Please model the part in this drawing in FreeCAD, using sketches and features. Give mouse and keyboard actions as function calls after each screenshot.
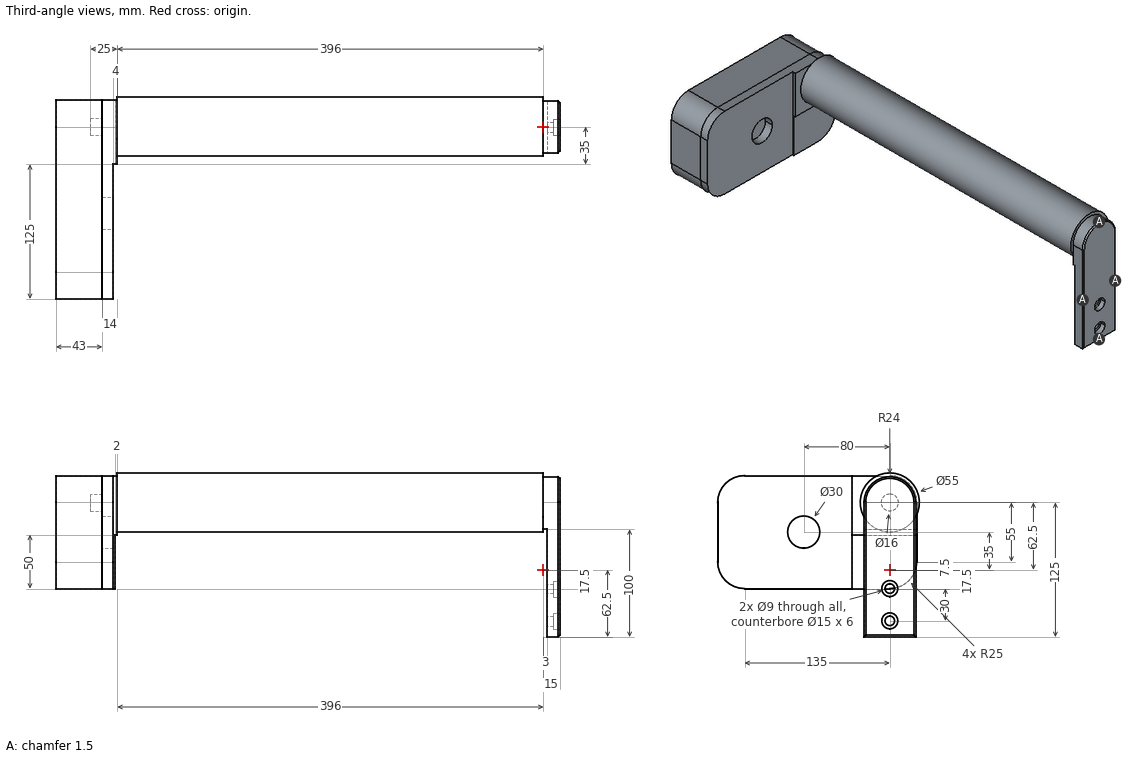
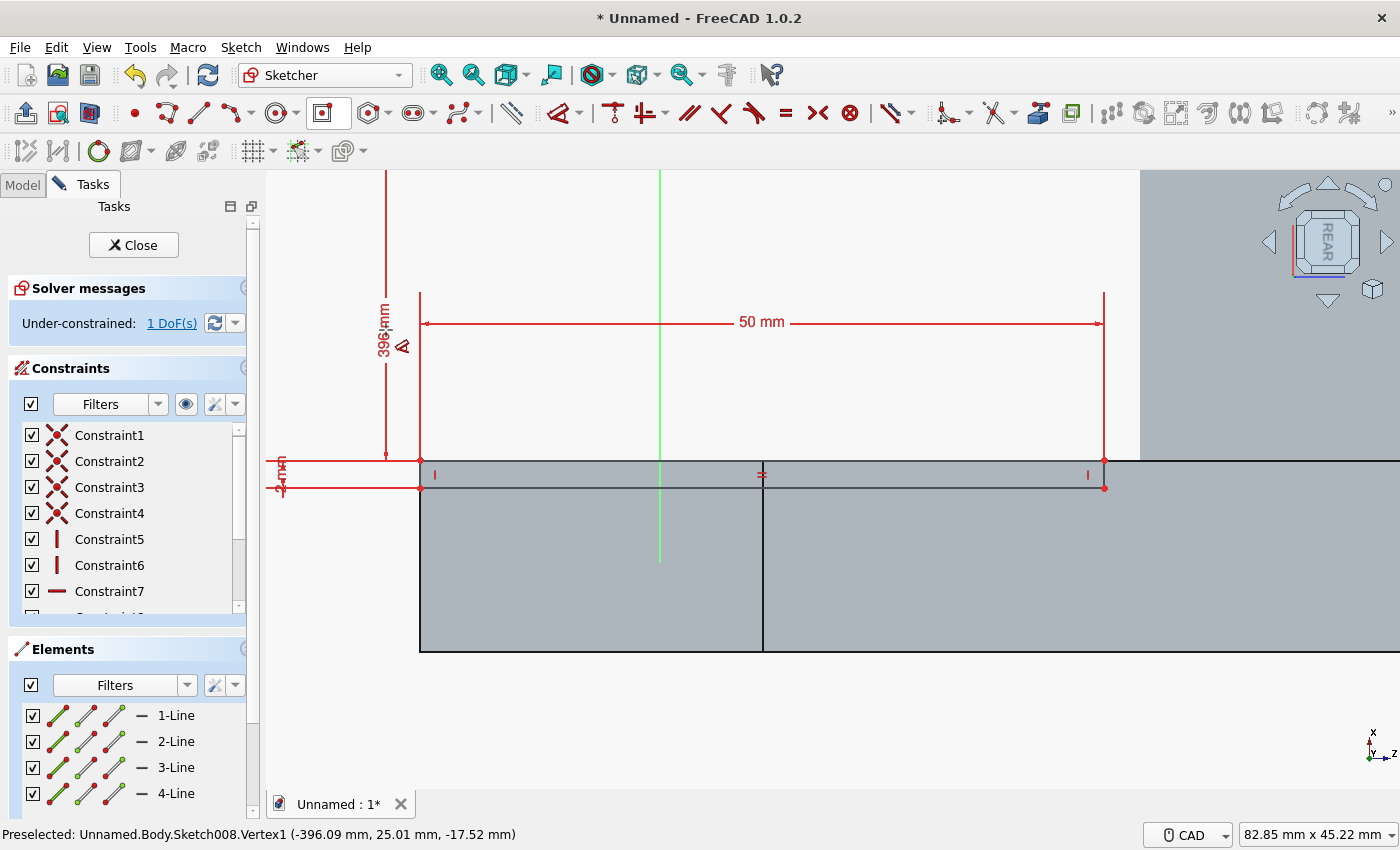
click(420, 461)
click(540, 519)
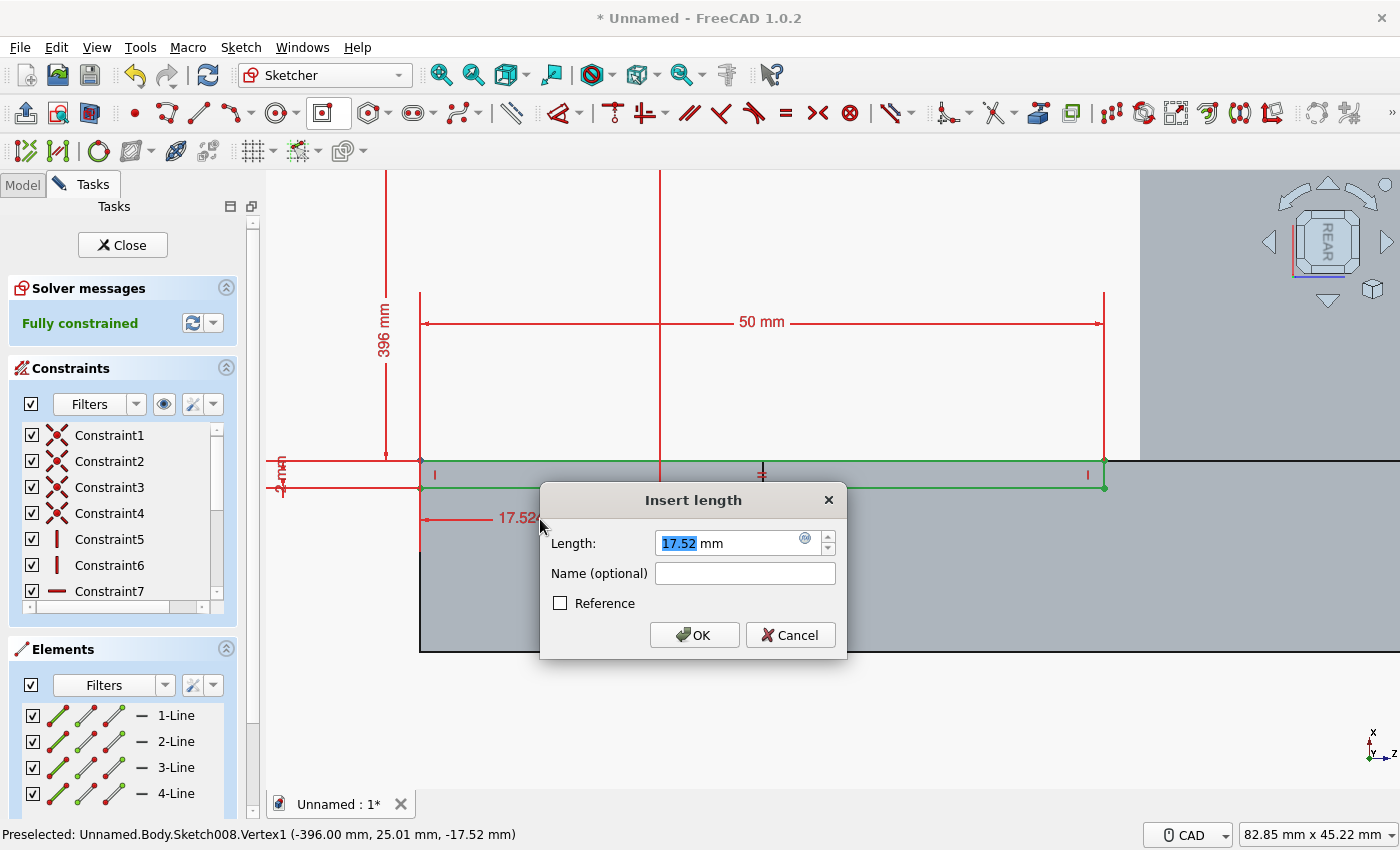
text(17.5)
key(Return)
key(Escape)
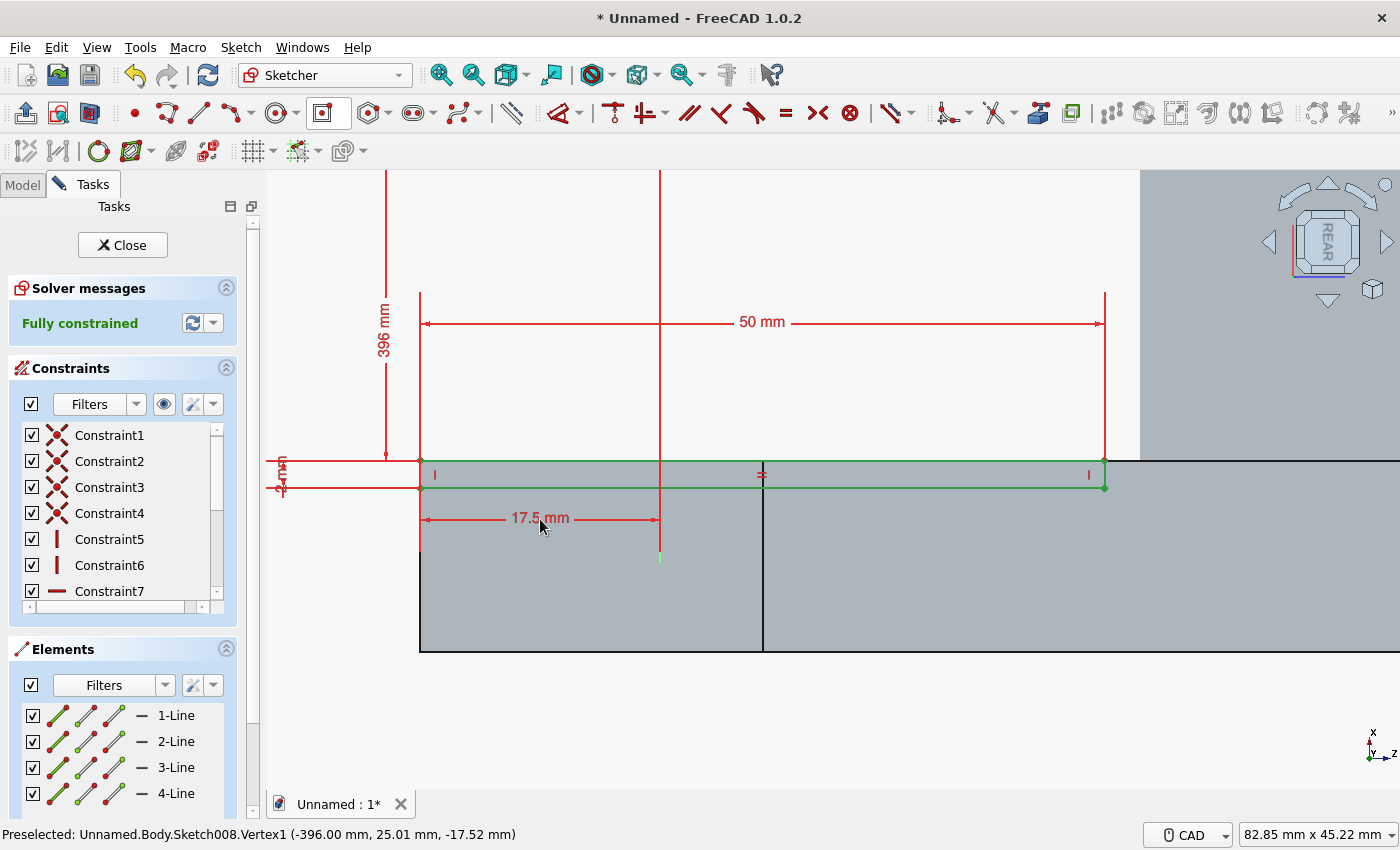
click(123, 245)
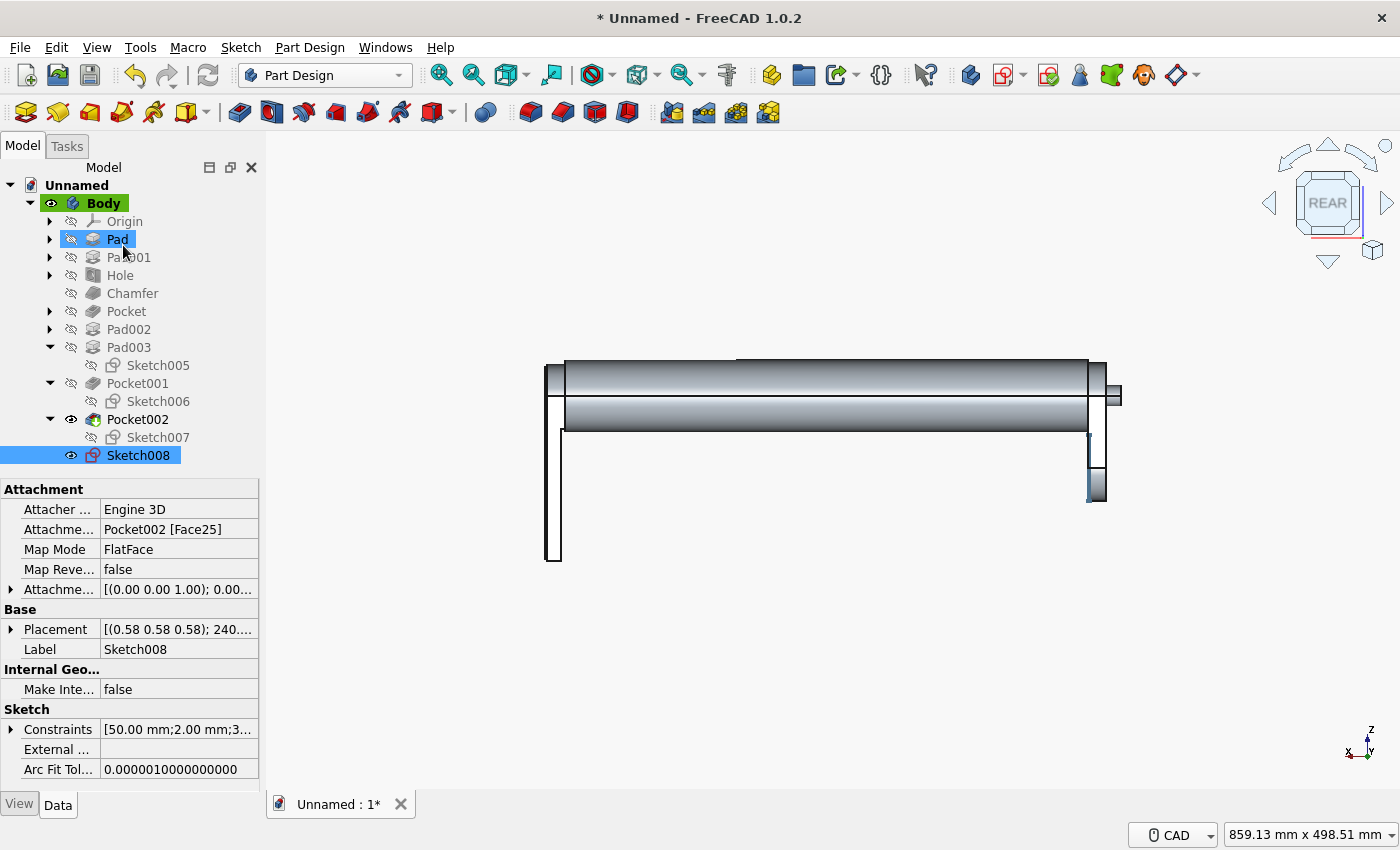
click(240, 112)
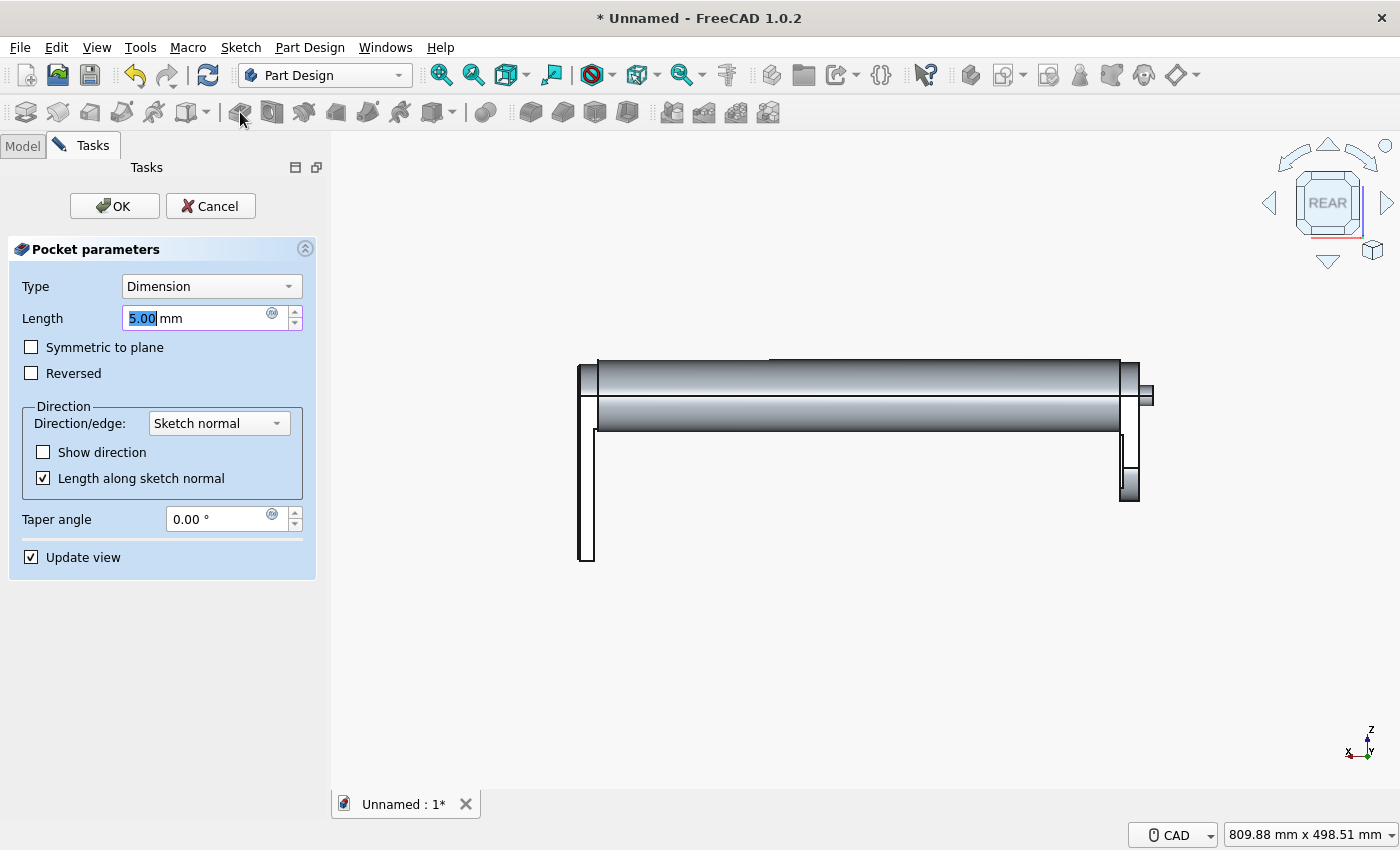
click(212, 286)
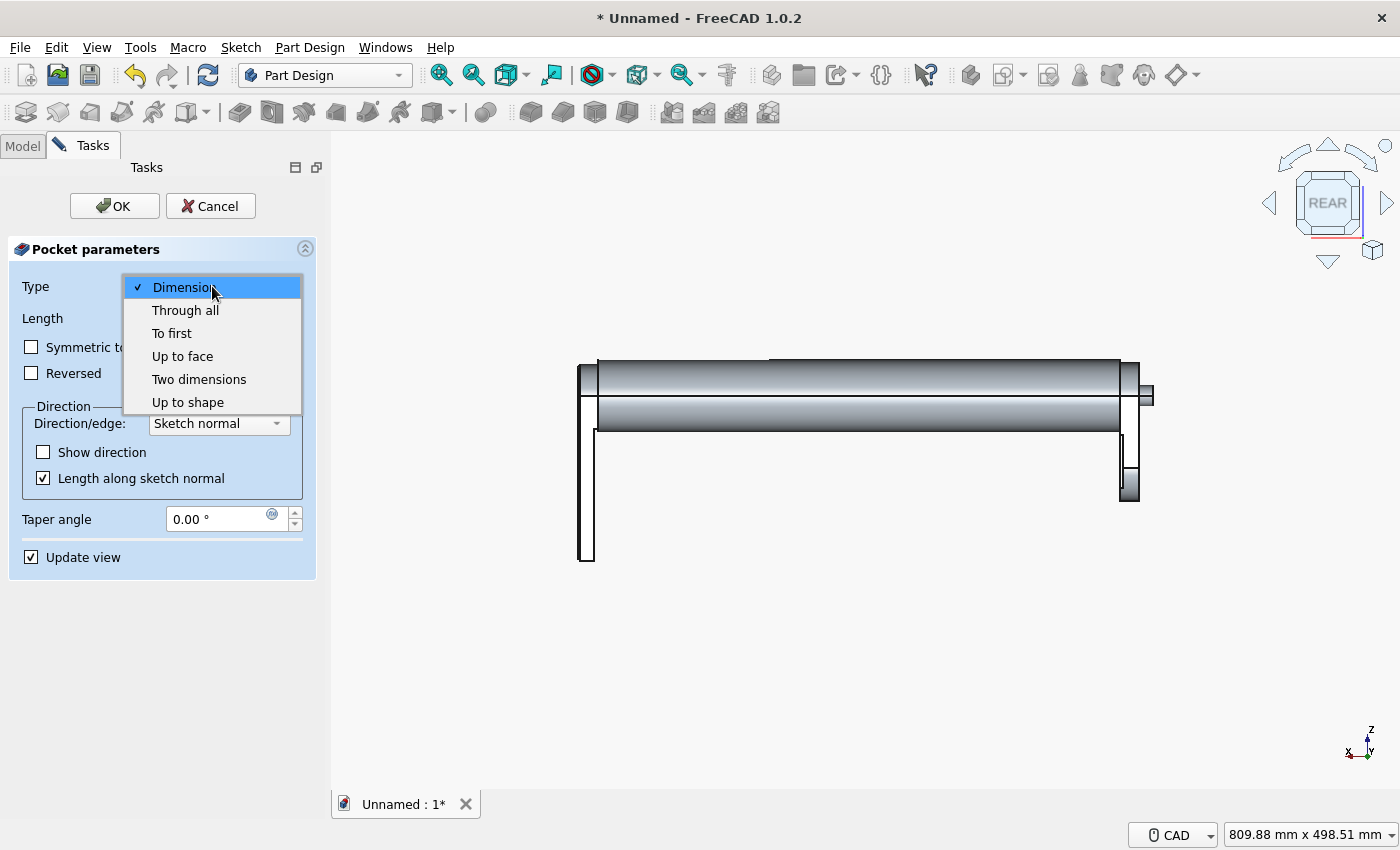
click(212, 310)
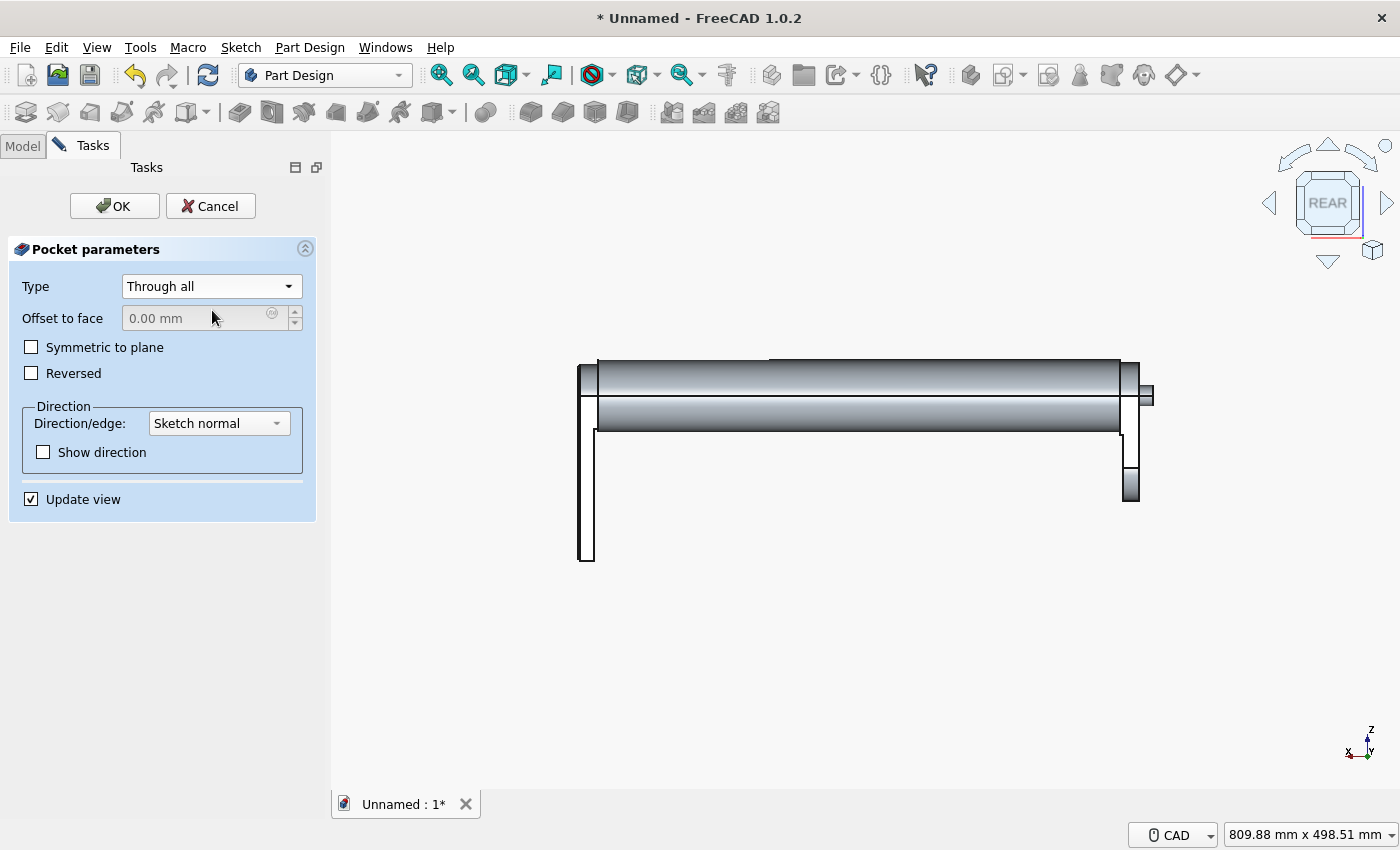
click(115, 206)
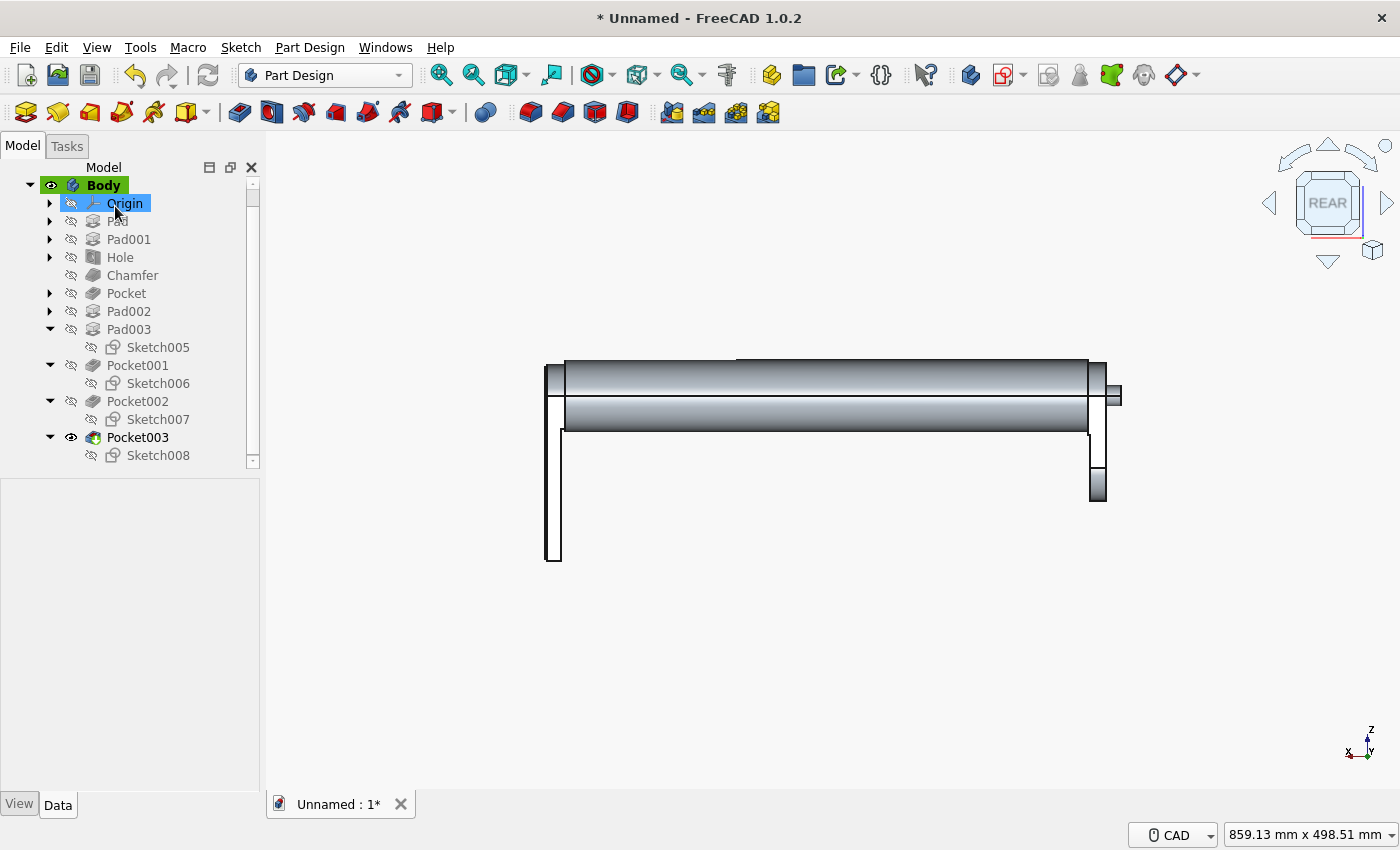
click(972, 76)